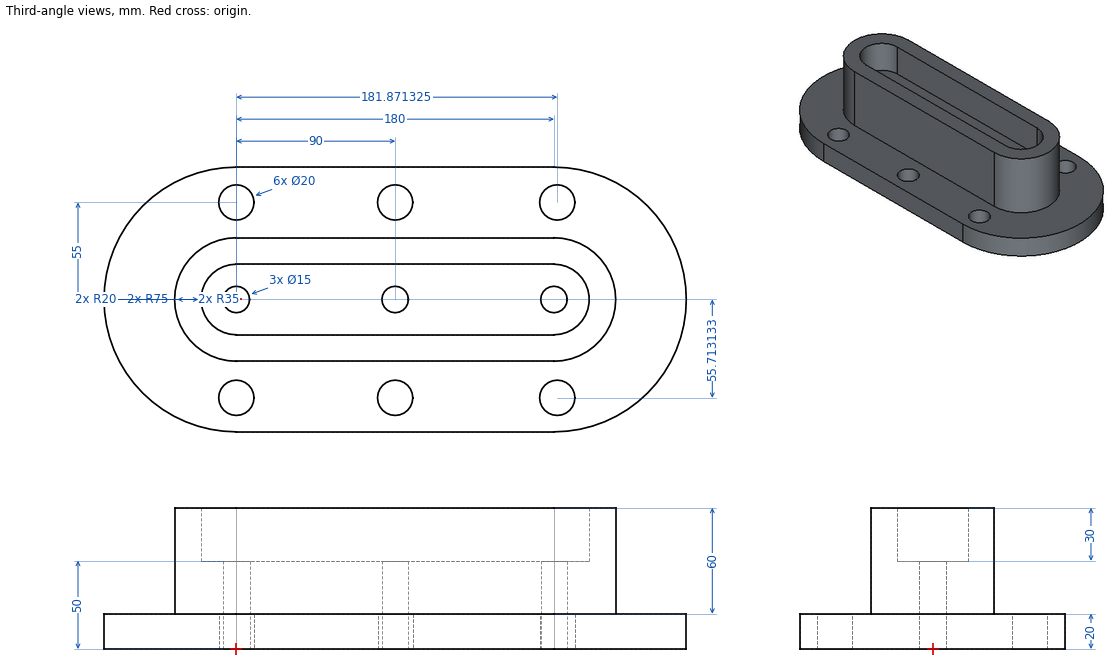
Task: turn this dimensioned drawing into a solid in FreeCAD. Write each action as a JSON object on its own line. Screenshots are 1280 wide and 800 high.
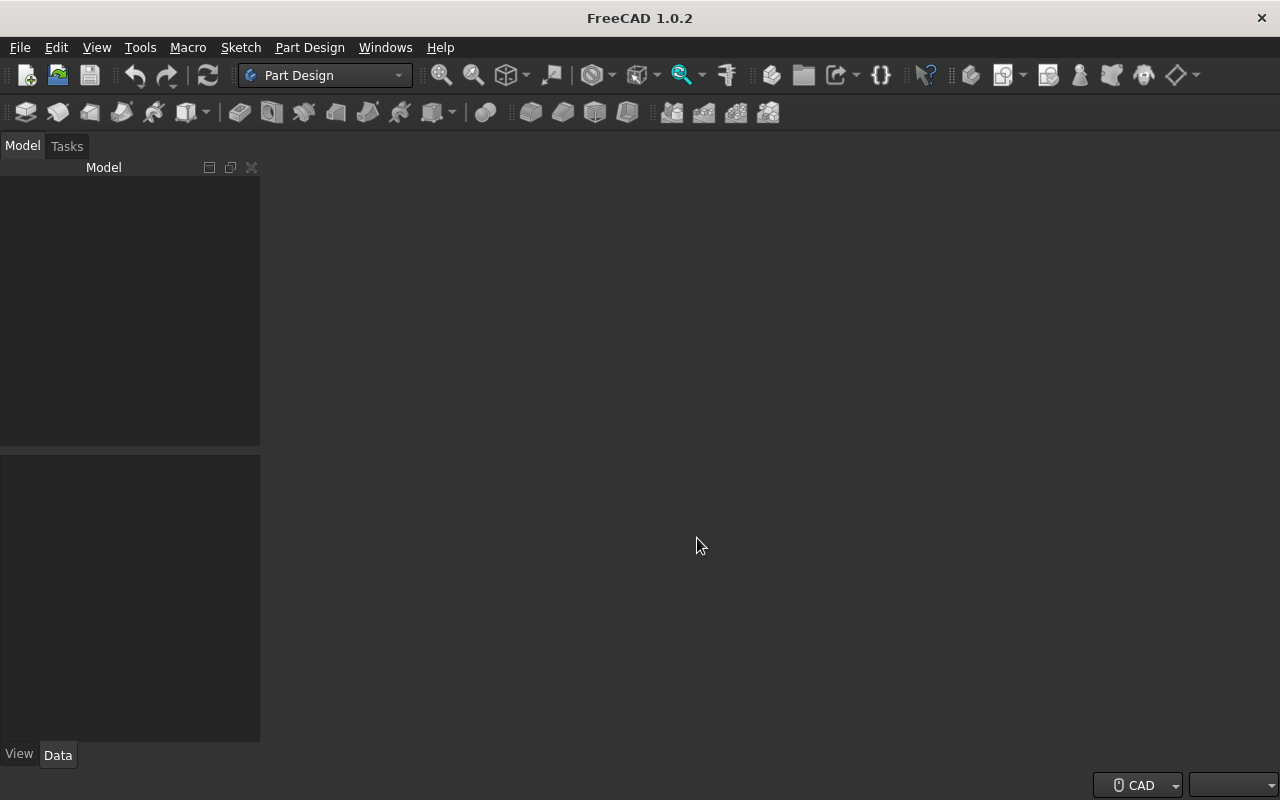
{"action": "left_click", "coordinate": [26, 76]}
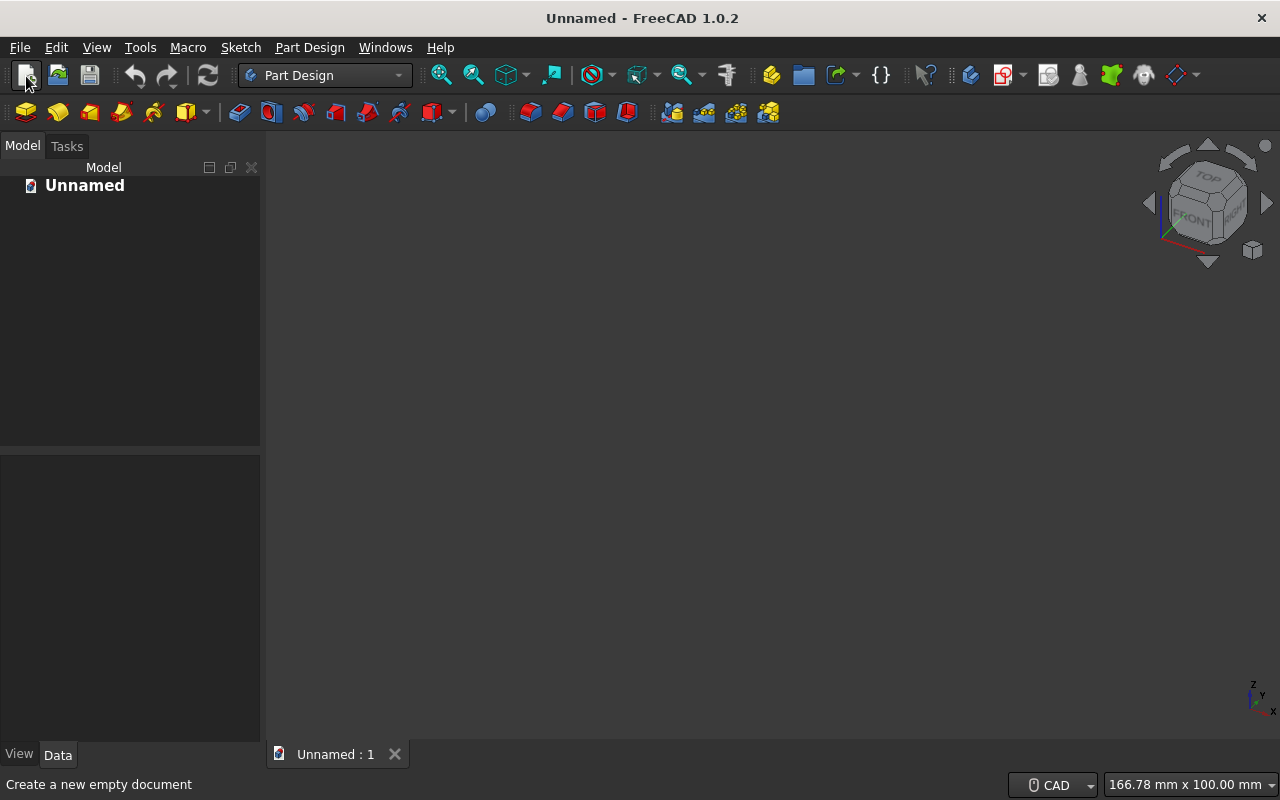
{"action": "left_click", "coordinate": [1004, 76]}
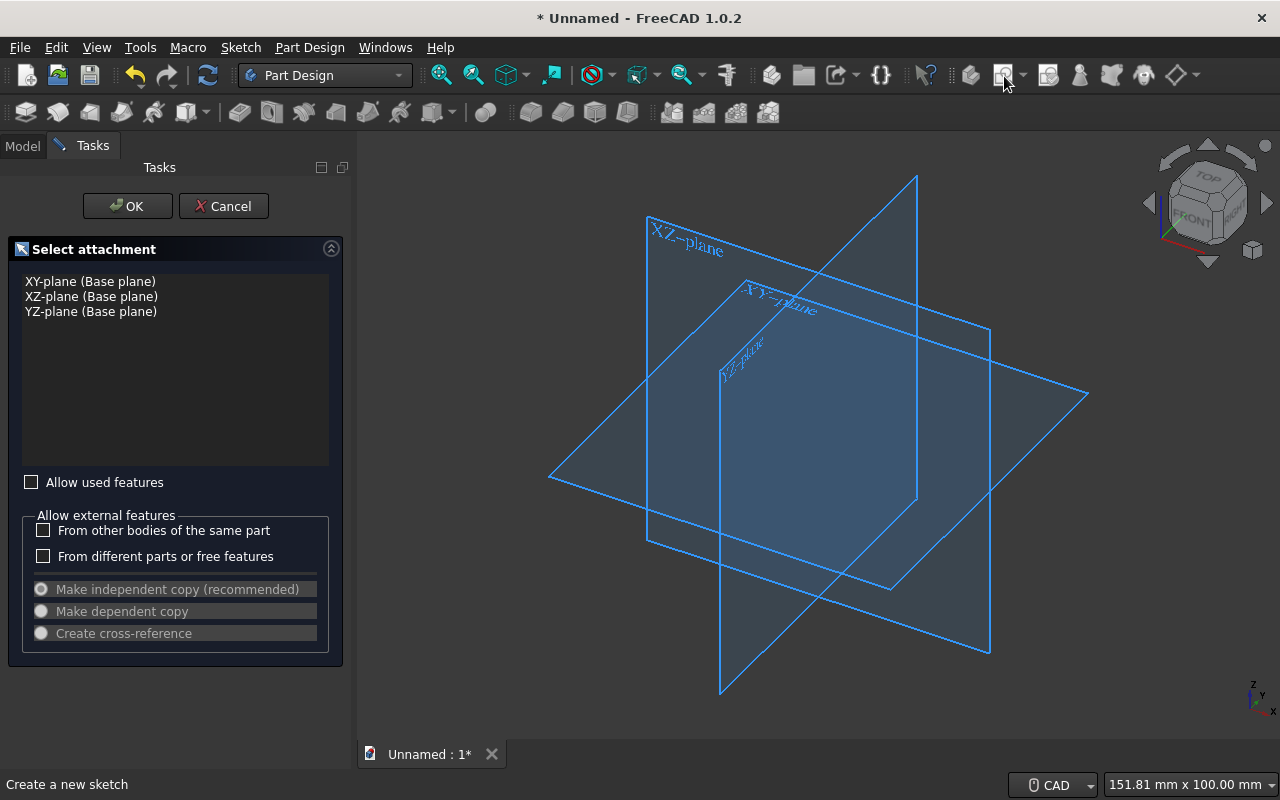
{"action": "left_click", "coordinate": [82, 282]}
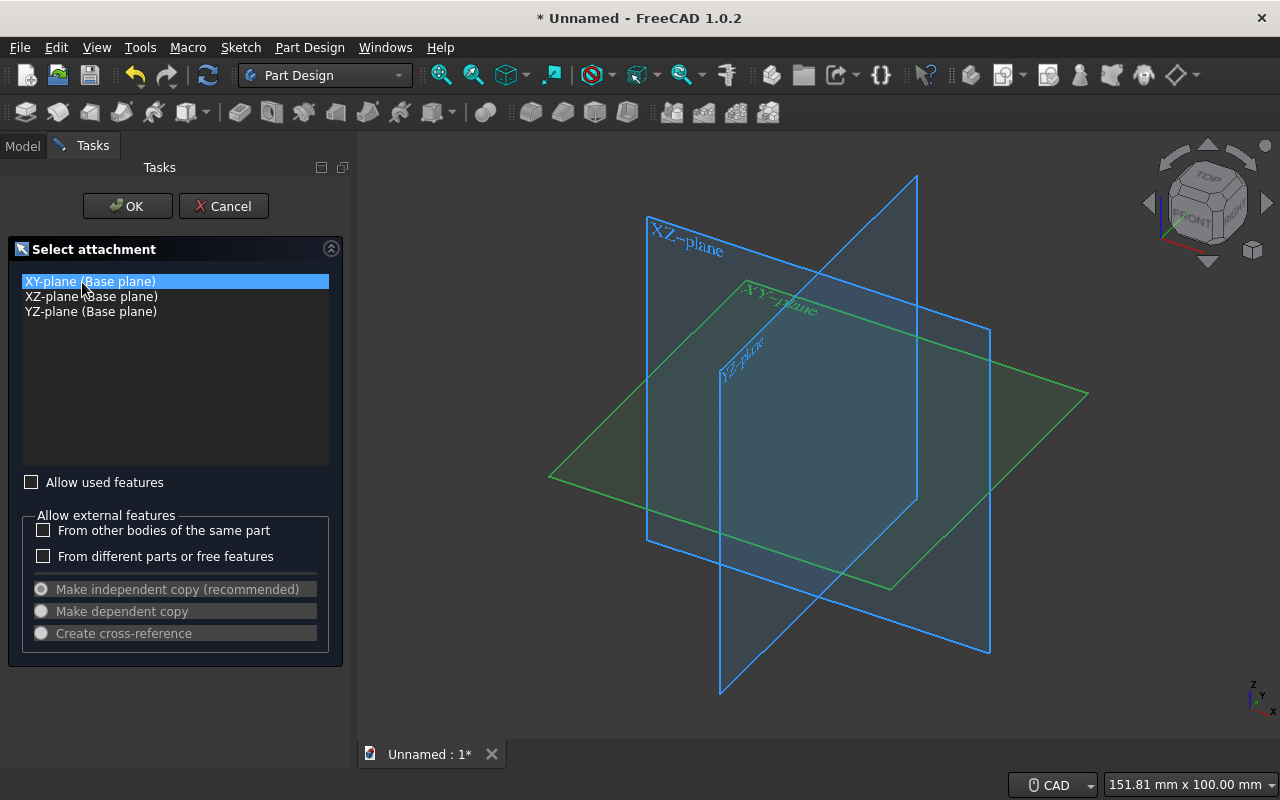
{"action": "left_click", "coordinate": [128, 206]}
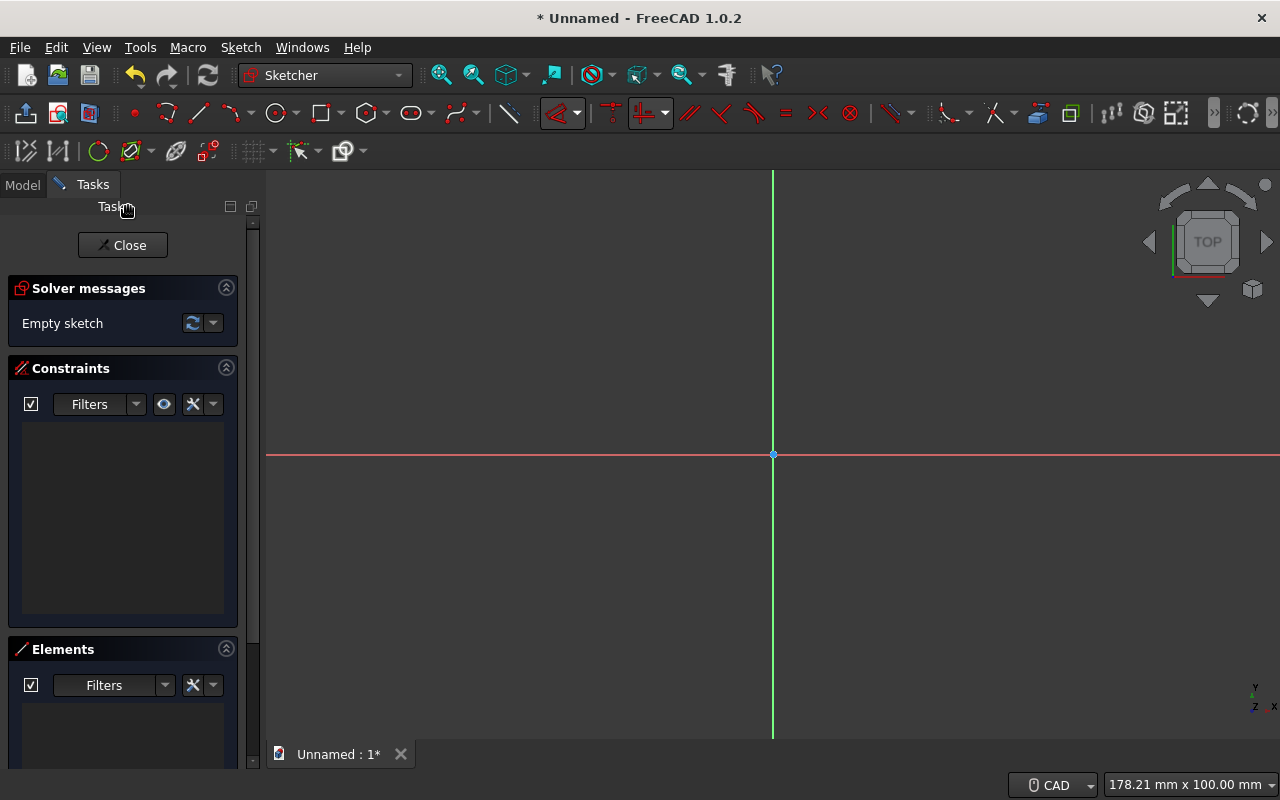
{"action": "scroll", "coordinate": [454, 454], "scroll_direction": "down", "scroll_amount": 6}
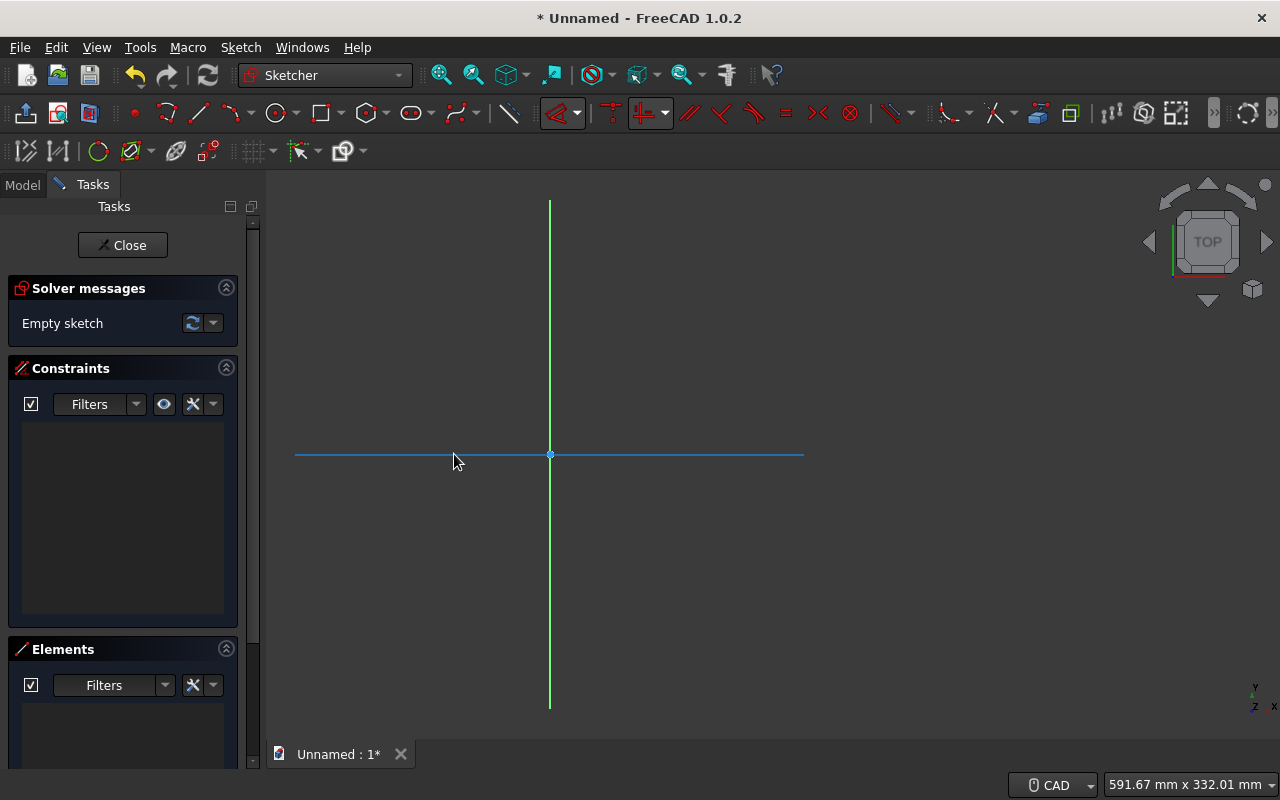
{"action": "left_click", "coordinate": [412, 114]}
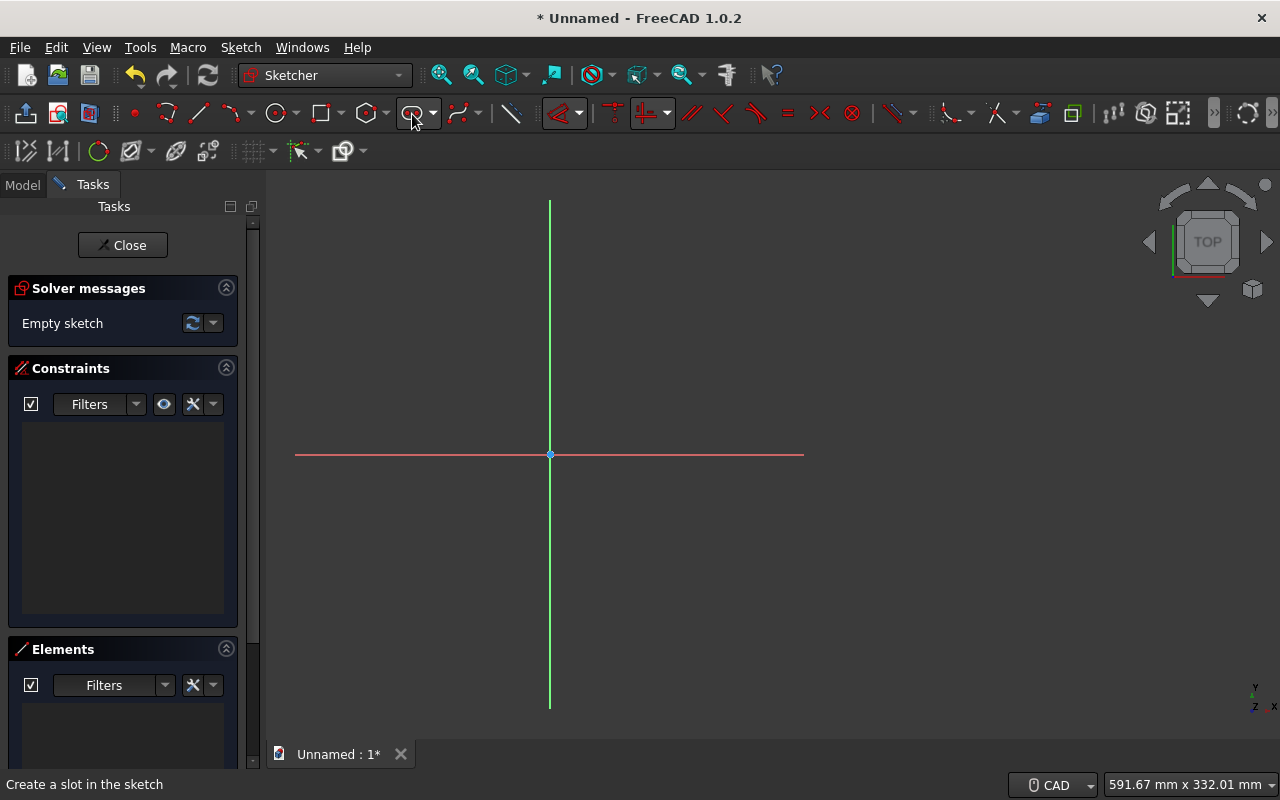
{"action": "left_click", "coordinate": [550, 454]}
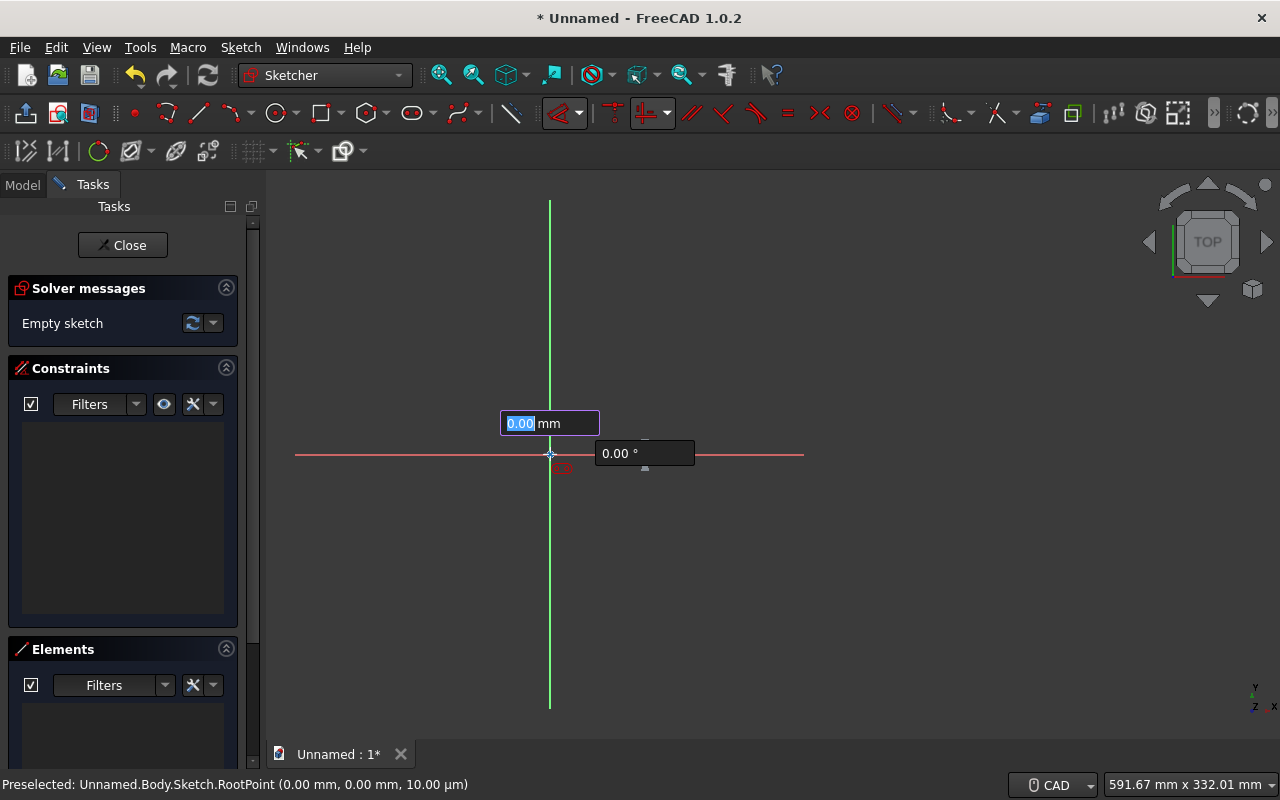
{"action": "left_click", "coordinate": [859, 446]}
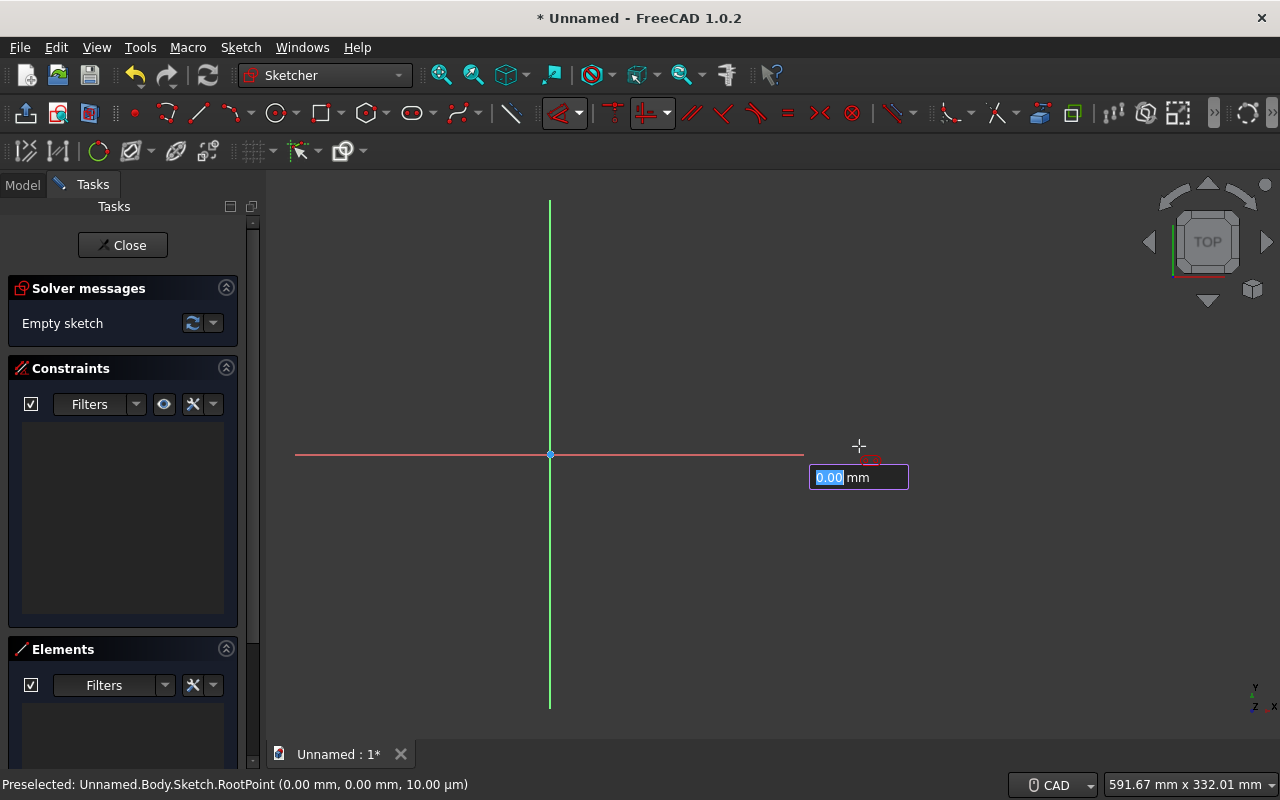
{"action": "left_click", "coordinate": [704, 326]}
{"action": "key", "text": "Escape"}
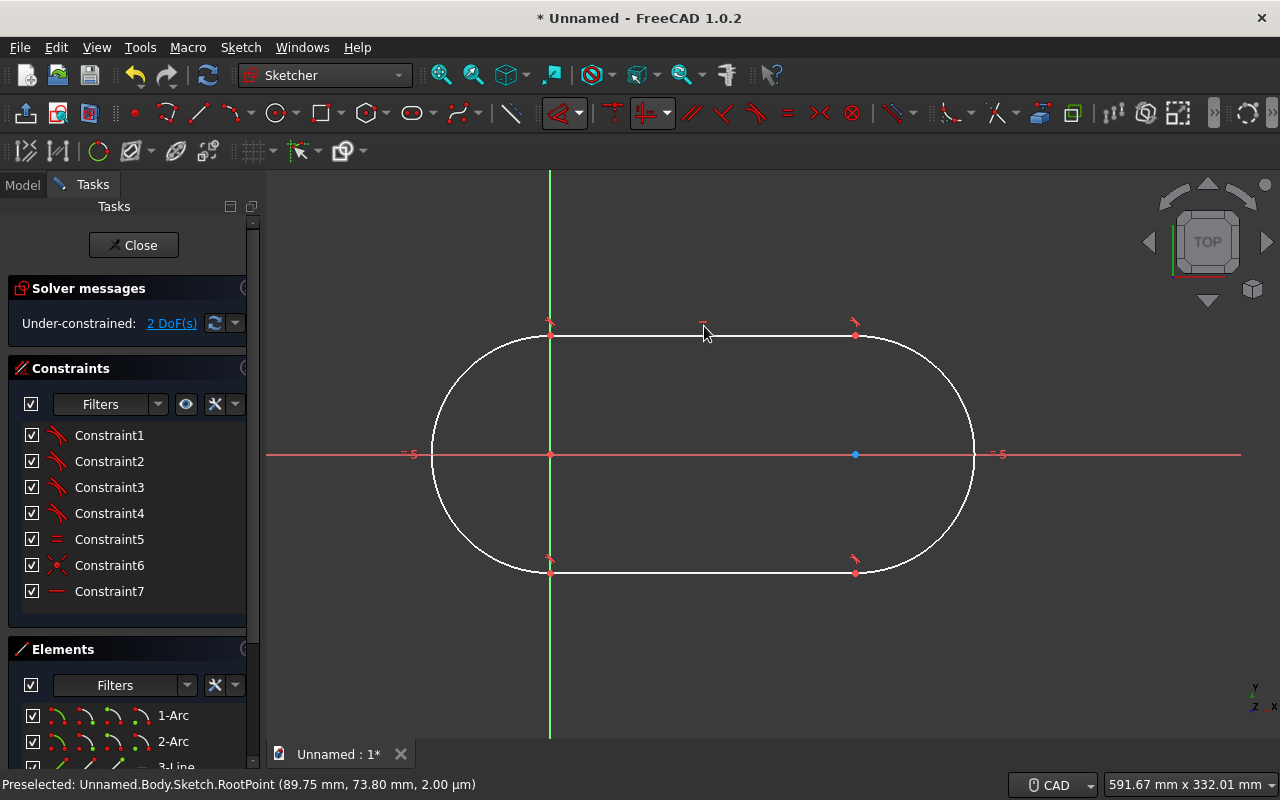
{"action": "left_click", "coordinate": [558, 114]}